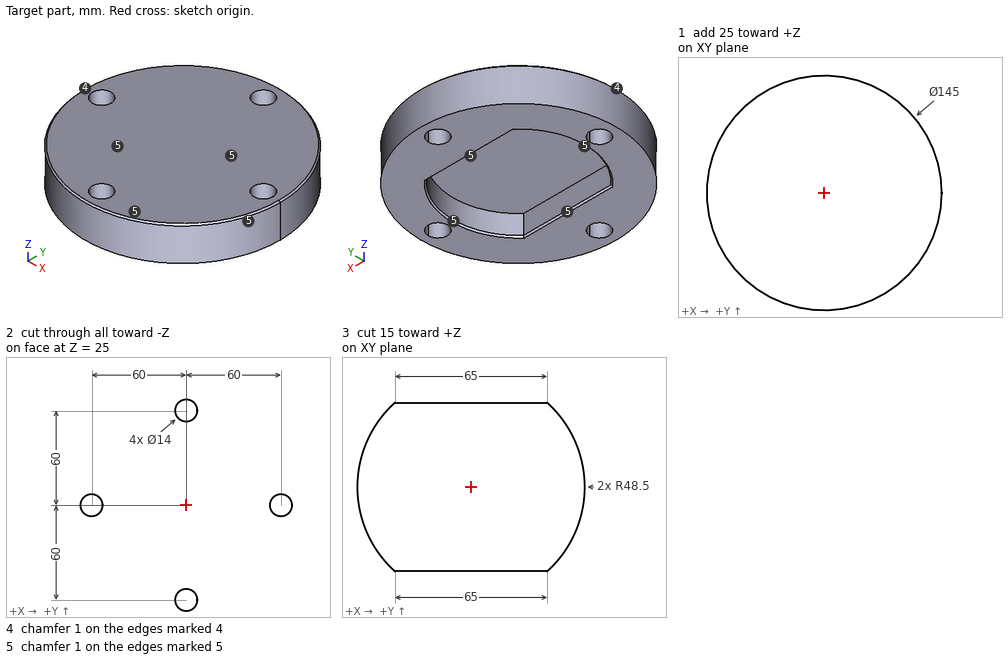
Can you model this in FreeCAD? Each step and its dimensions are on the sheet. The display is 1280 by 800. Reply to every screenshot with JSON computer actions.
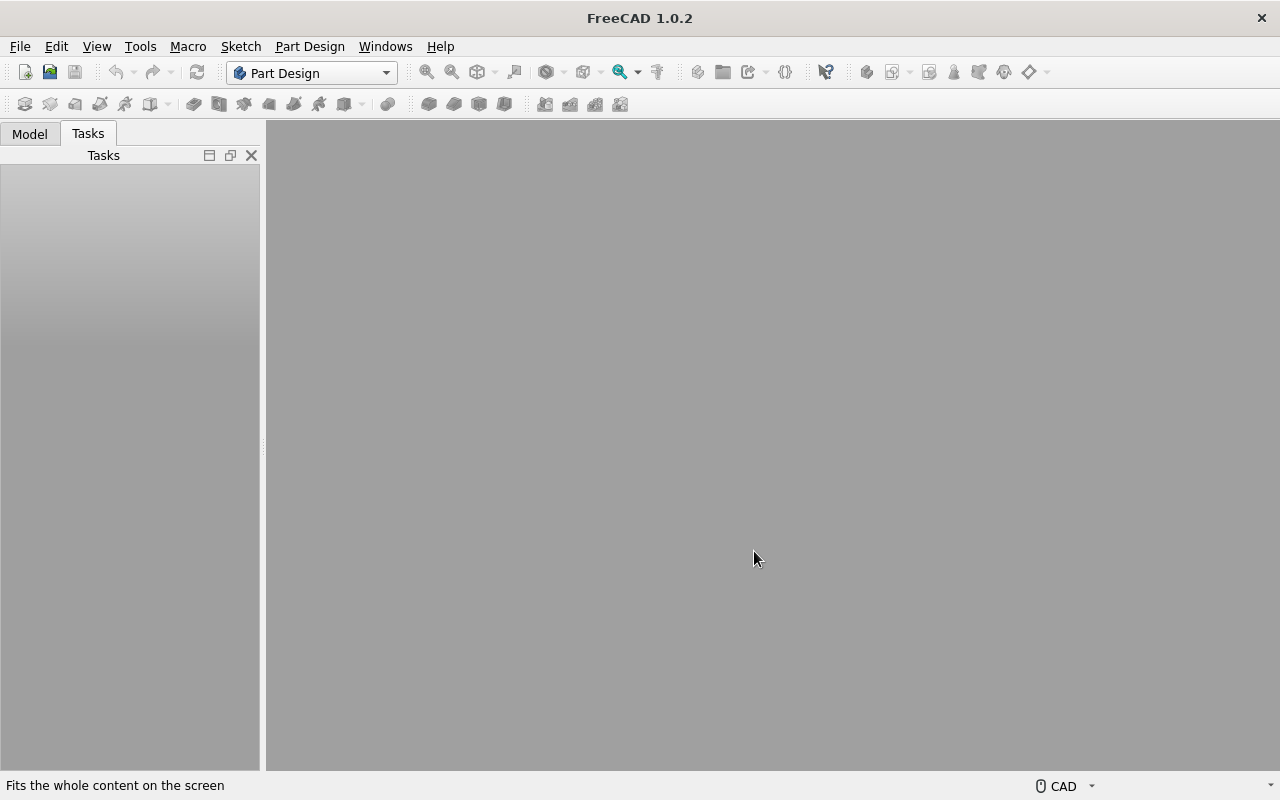
{"action": "left_click", "coordinate": [25, 72]}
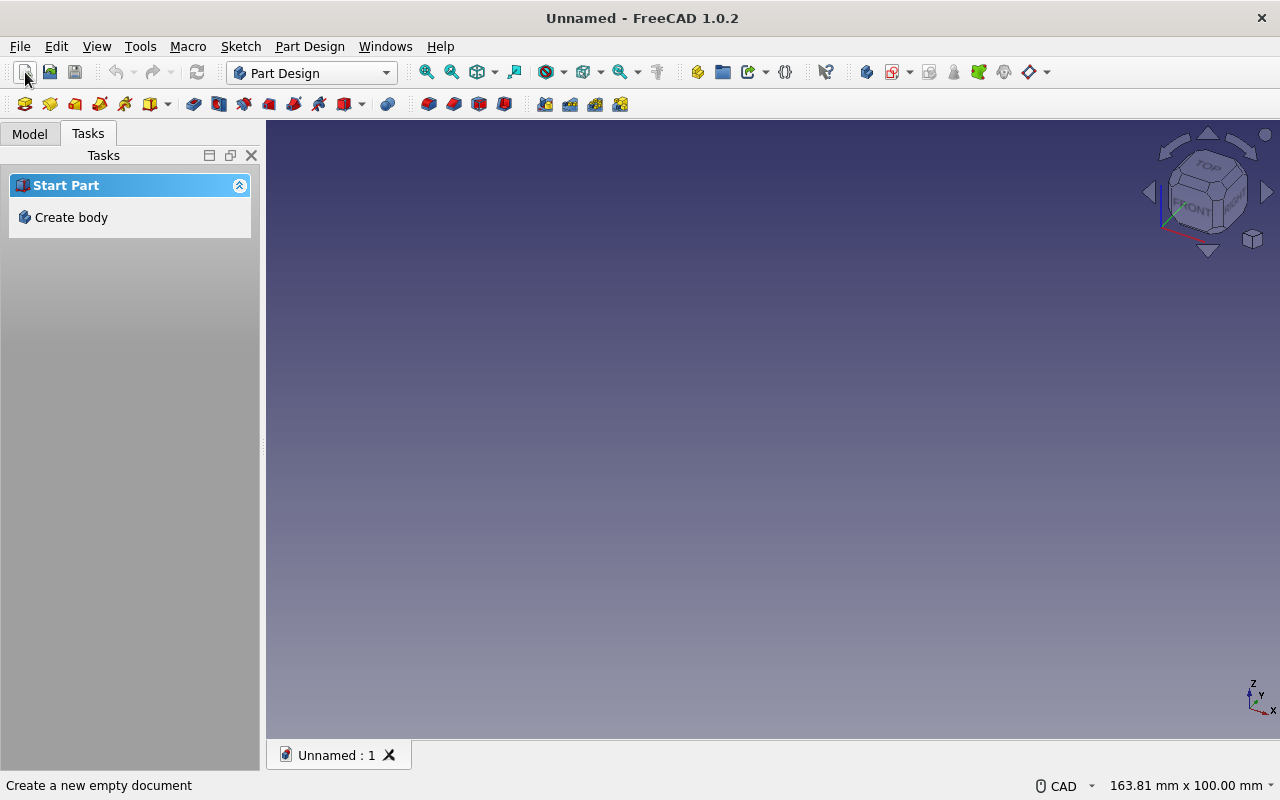
{"action": "left_click", "coordinate": [892, 72]}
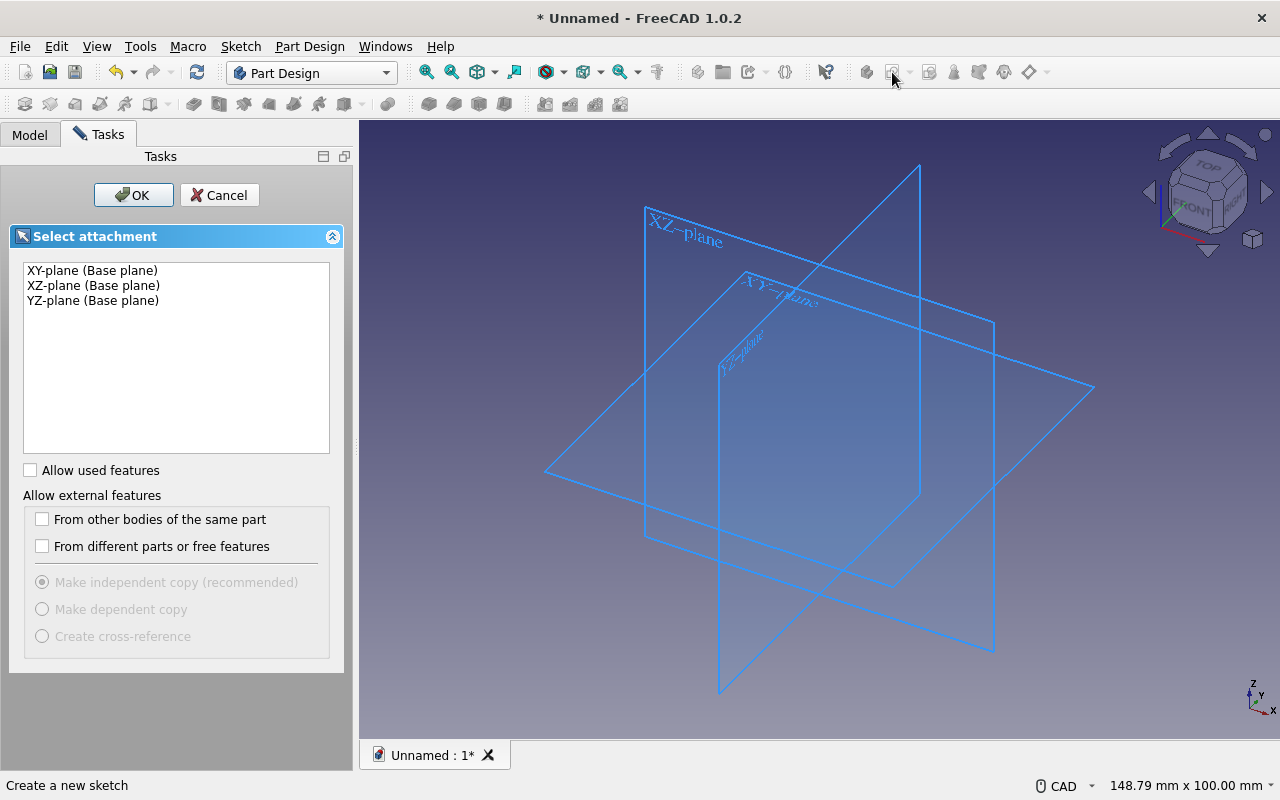
{"action": "left_click", "coordinate": [84, 270]}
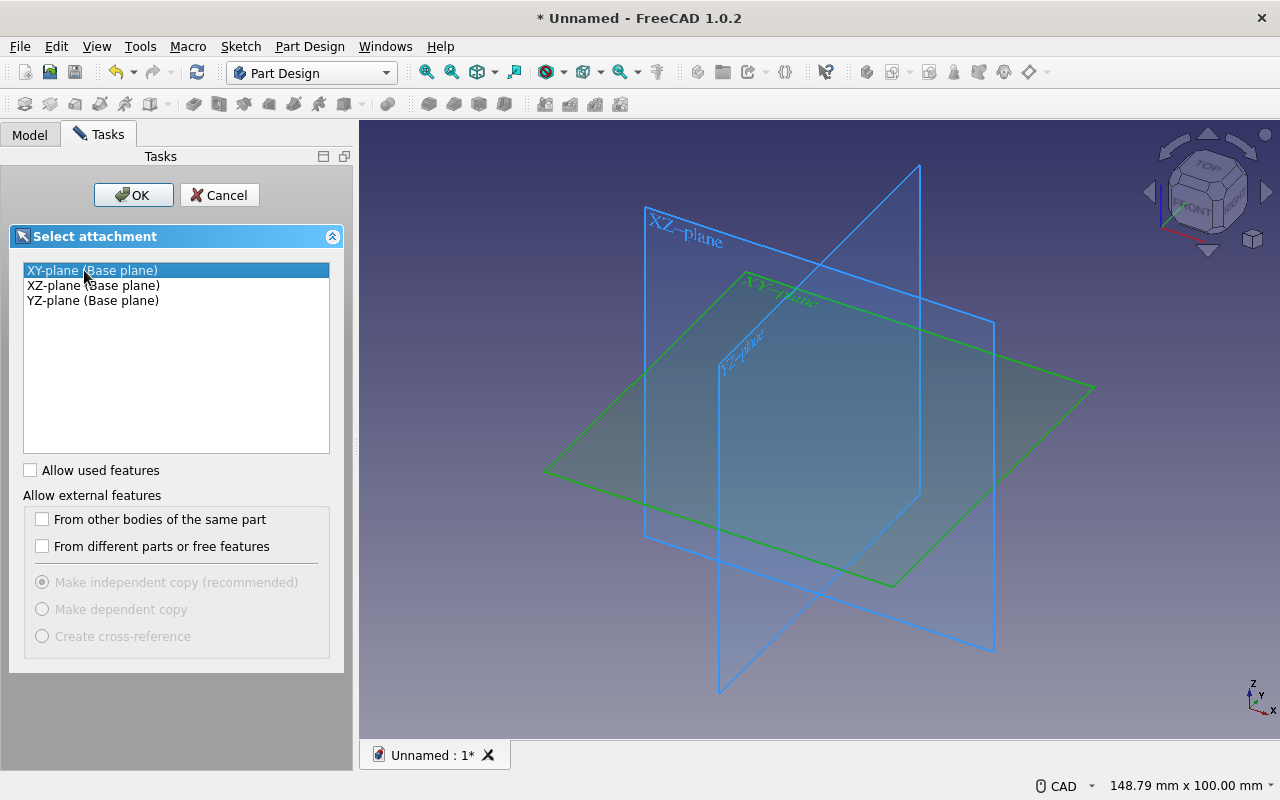
{"action": "left_click", "coordinate": [134, 195]}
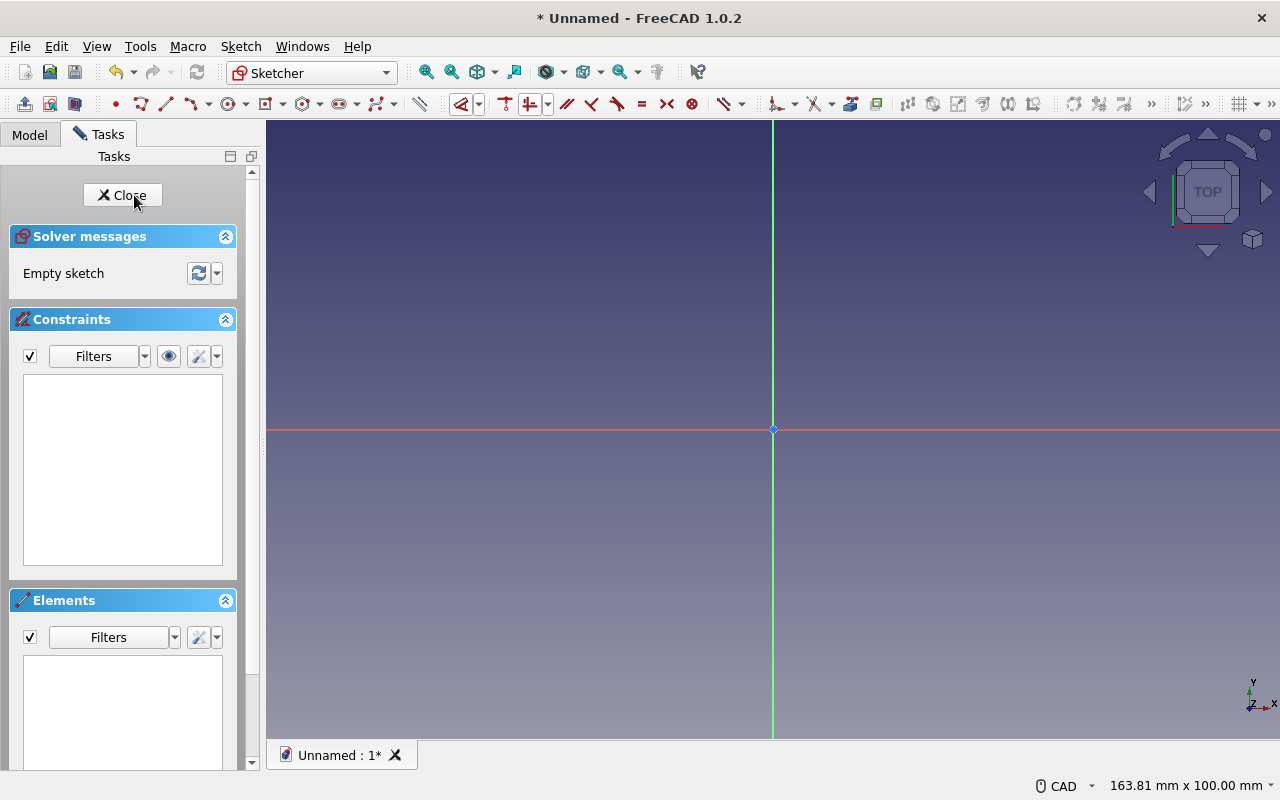
{"action": "scroll", "coordinate": [649, 430], "scroll_direction": "down", "scroll_amount": 4}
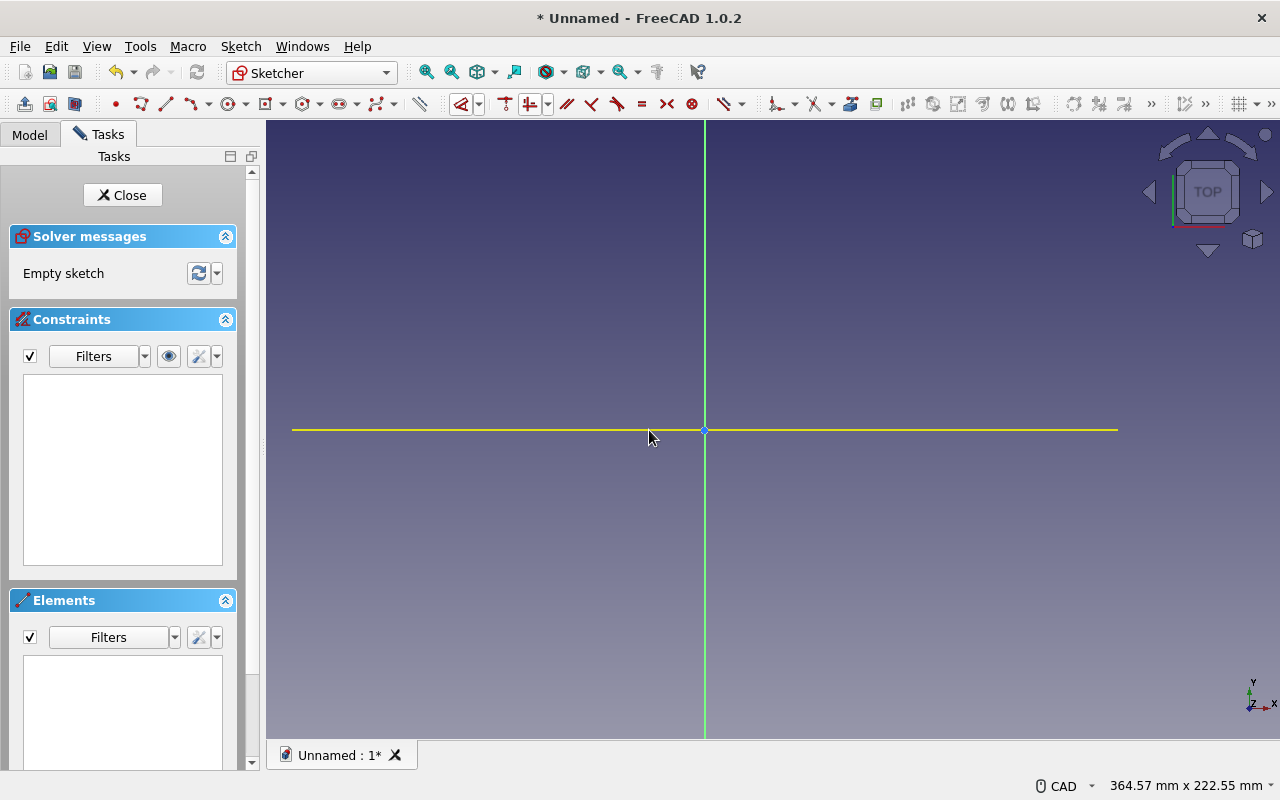
{"action": "left_click", "coordinate": [228, 104]}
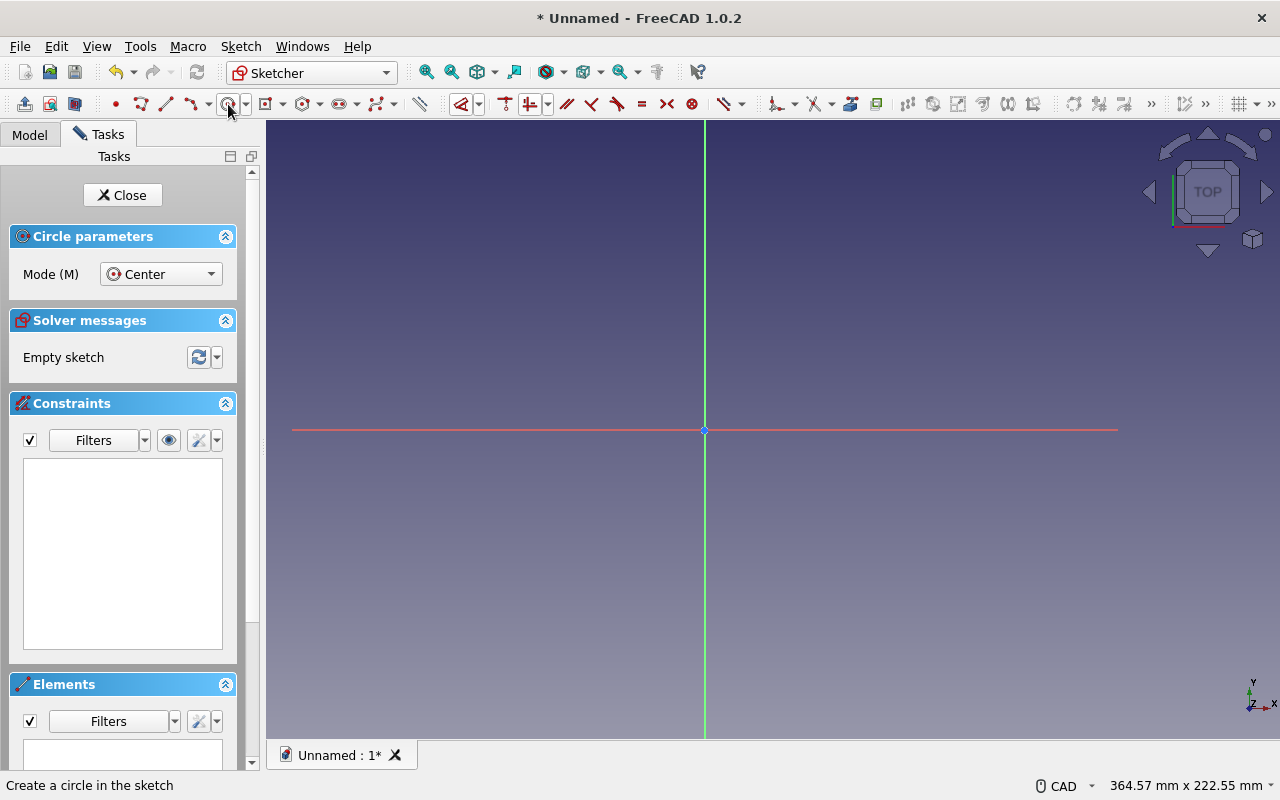
{"action": "left_click", "coordinate": [705, 430]}
{"action": "left_click", "coordinate": [848, 287]}
{"action": "key", "text": "Escape"}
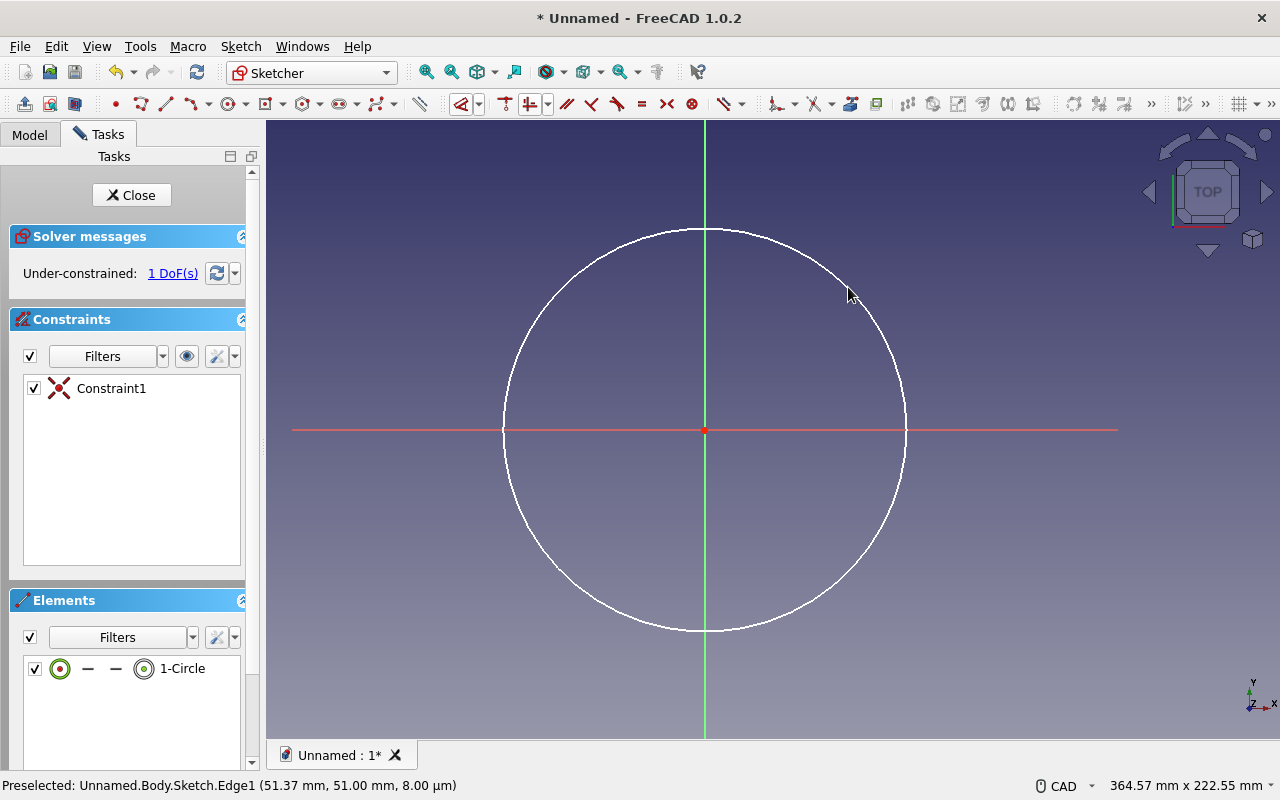
{"action": "left_click", "coordinate": [847, 287]}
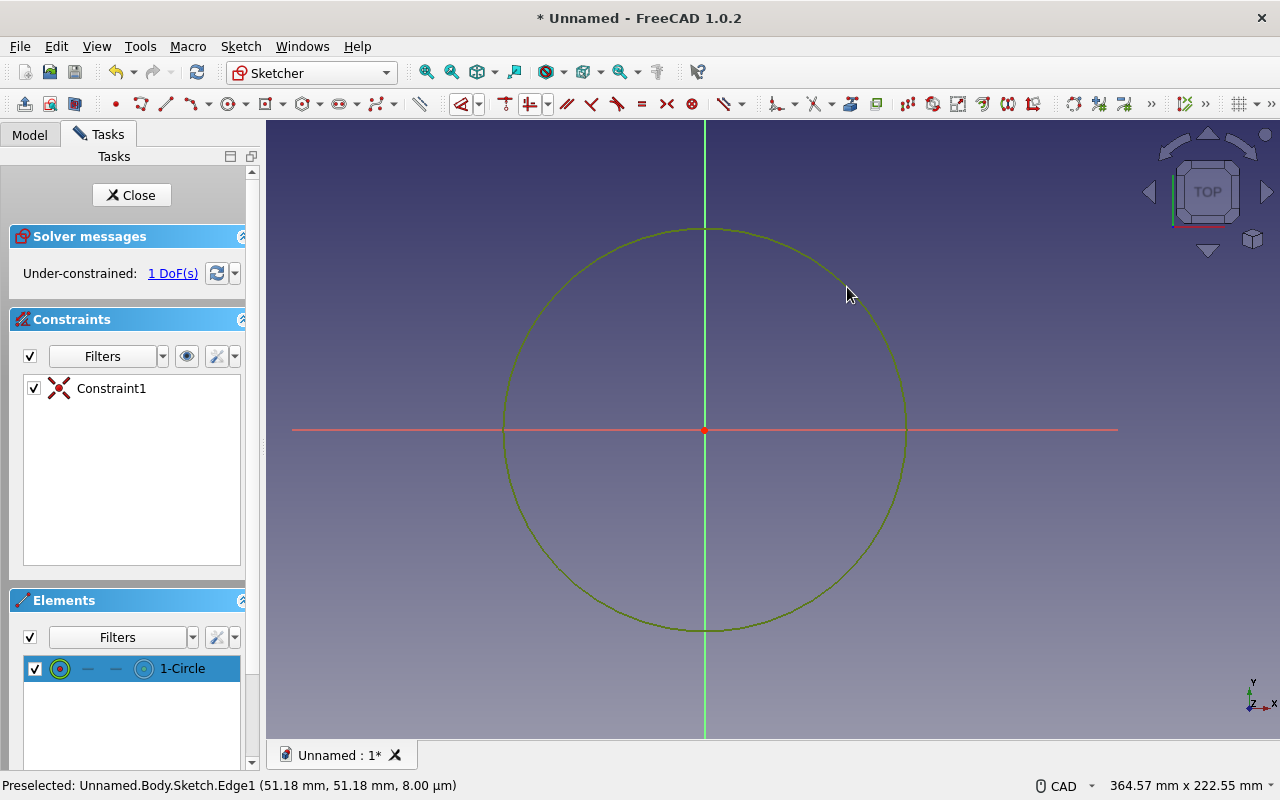
{"action": "left_click", "coordinate": [478, 104]}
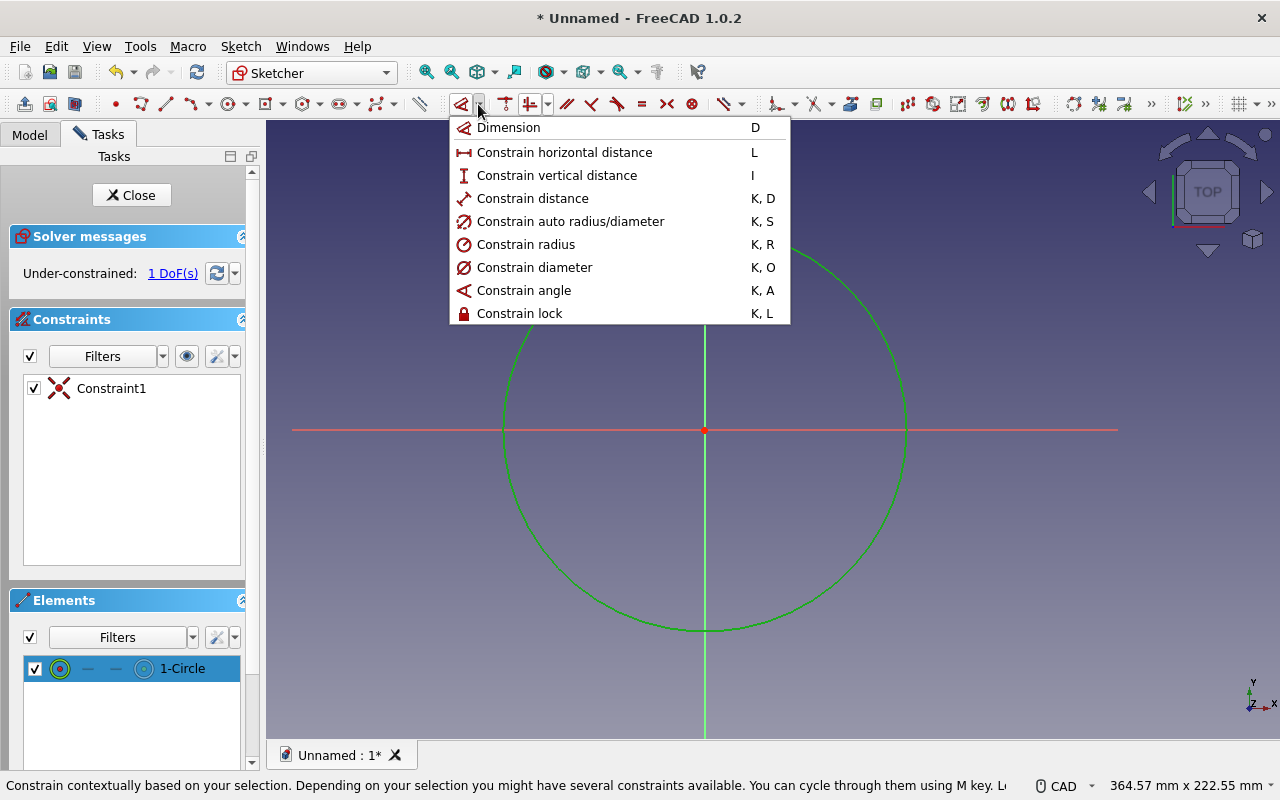
{"action": "left_click", "coordinate": [620, 268]}